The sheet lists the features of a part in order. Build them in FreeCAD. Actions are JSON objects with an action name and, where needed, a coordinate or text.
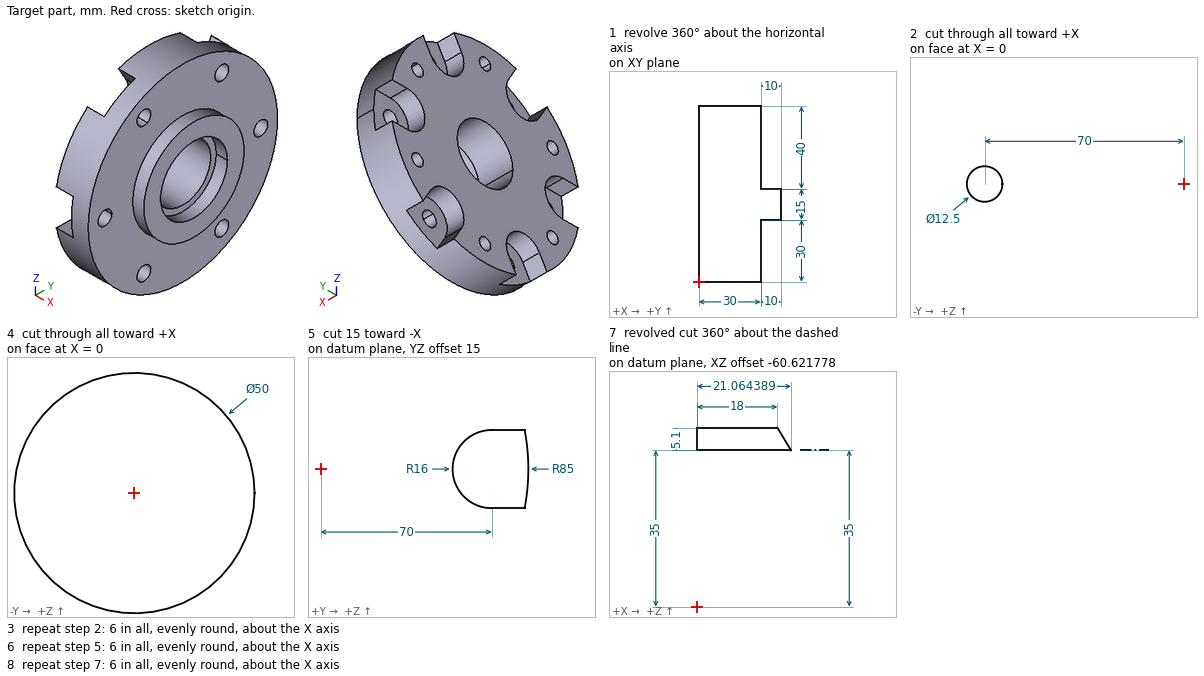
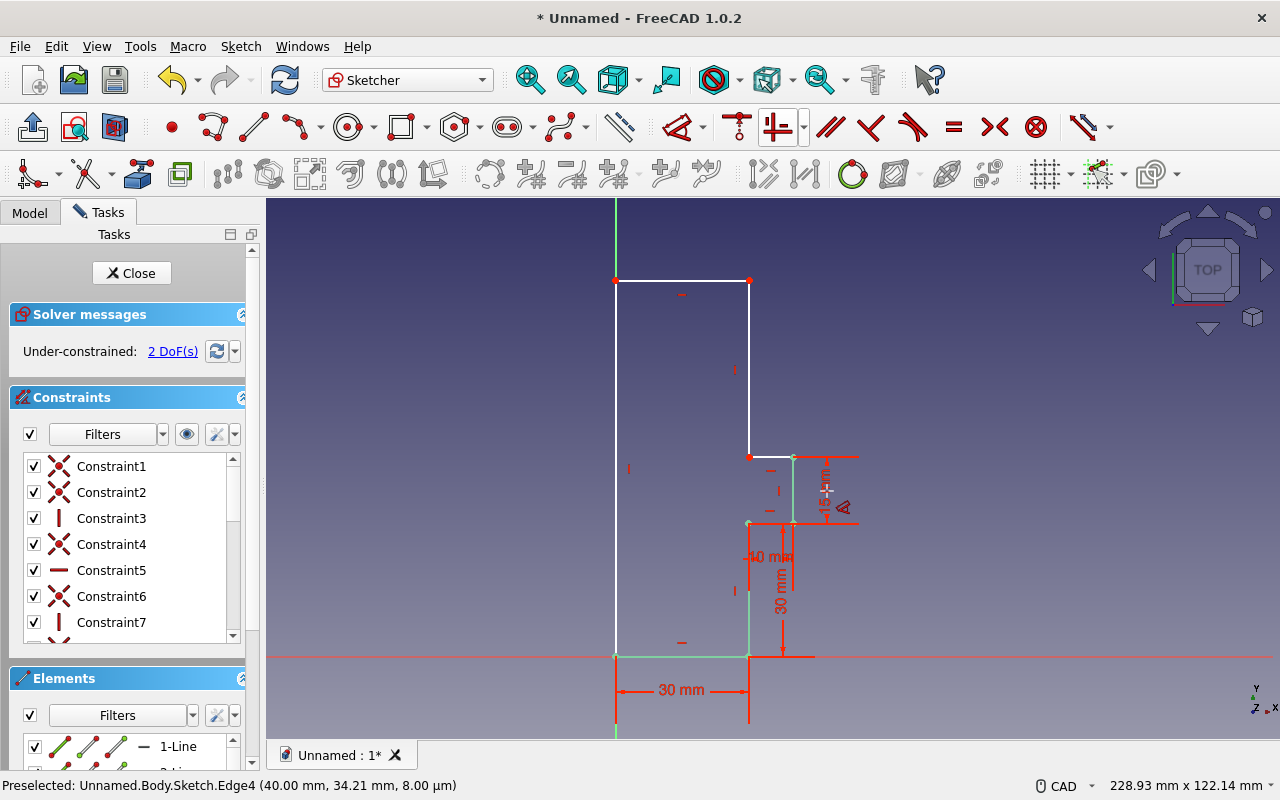
{"action": "left_click", "coordinate": [780, 457]}
{"action": "left_click", "coordinate": [771, 423]}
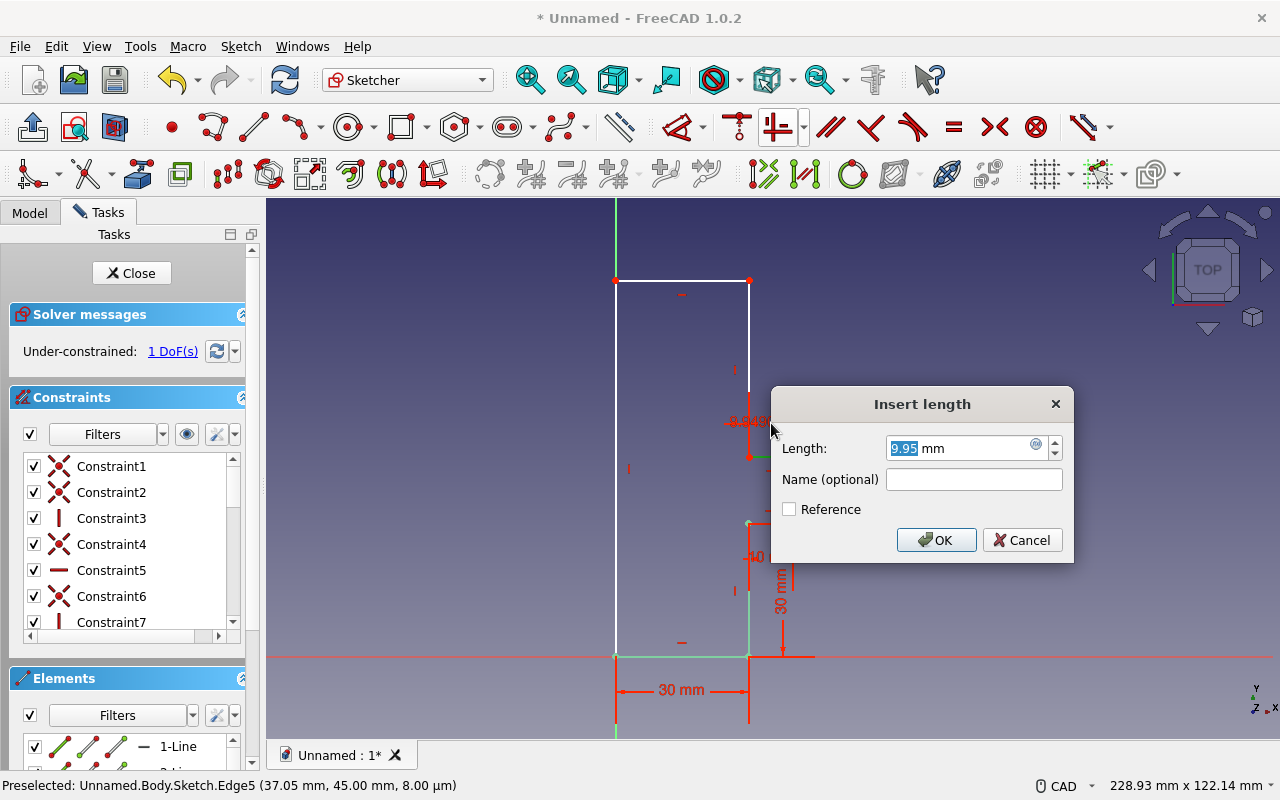
{"action": "type", "text": "10"}
{"action": "key", "text": "Return"}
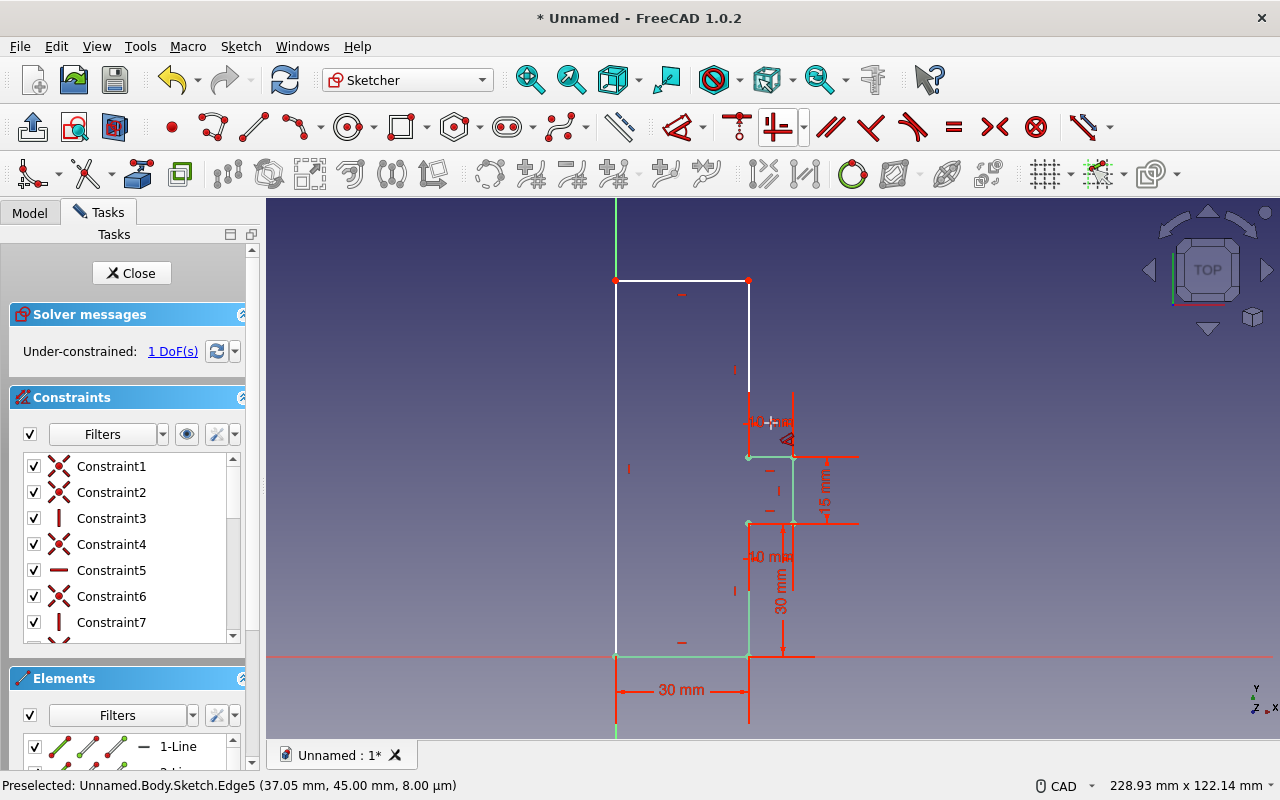
{"action": "left_click", "coordinate": [749, 404]}
{"action": "left_click", "coordinate": [783, 369]}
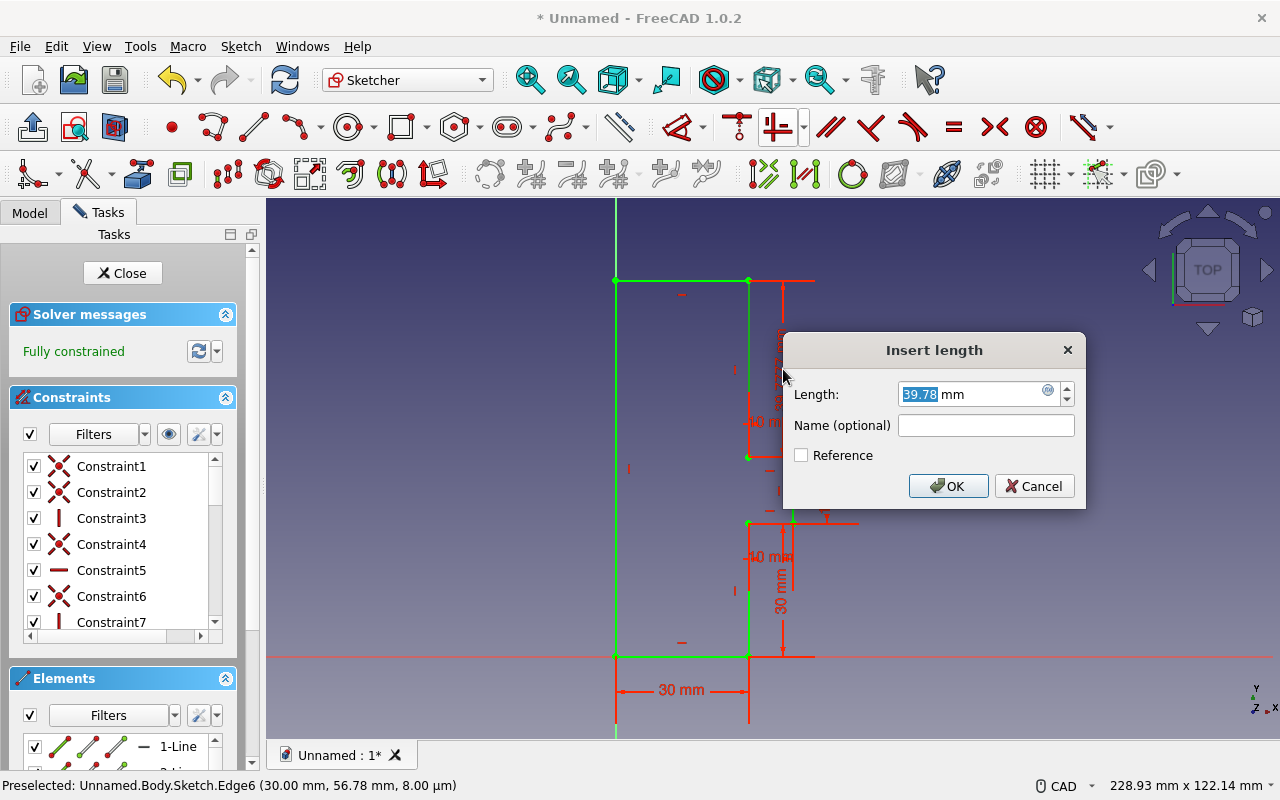
{"action": "type", "text": "40"}
{"action": "key", "text": "Return"}
{"action": "key", "text": "Escape"}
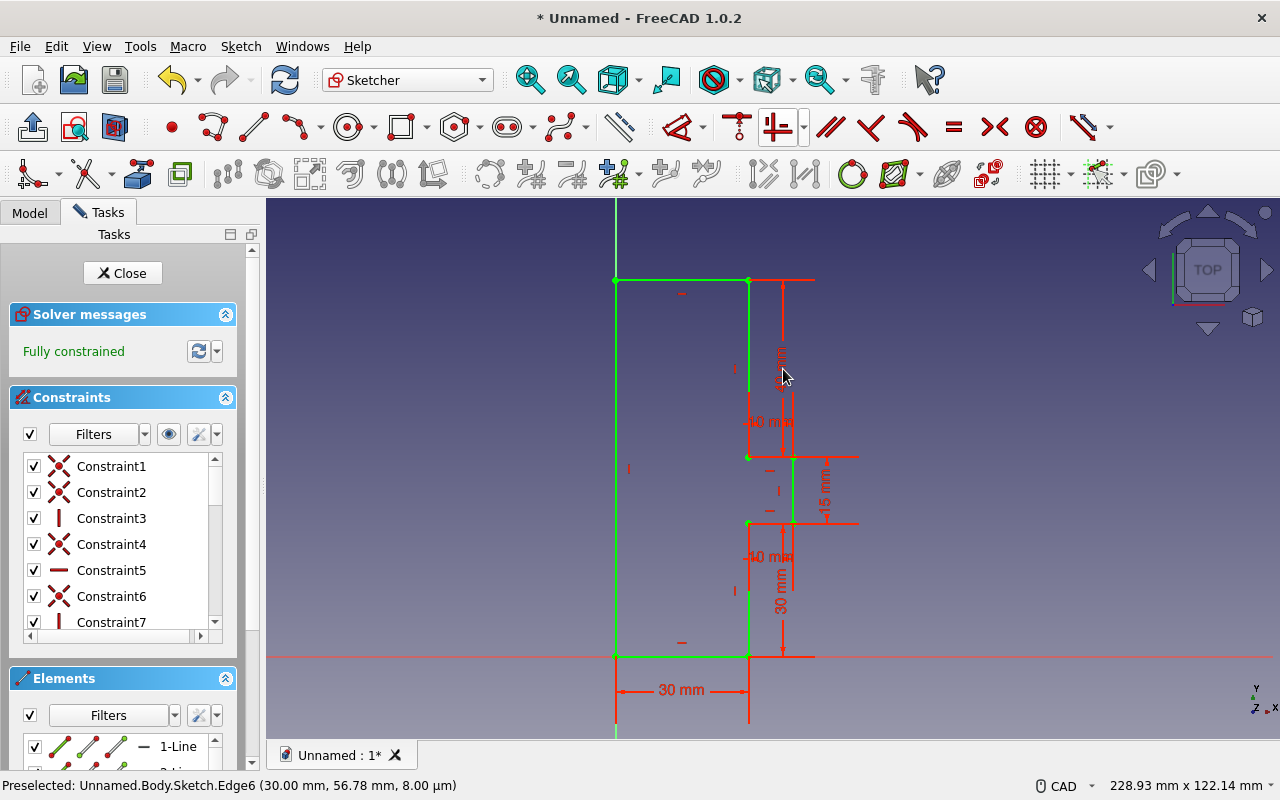
{"action": "left_click", "coordinate": [123, 273]}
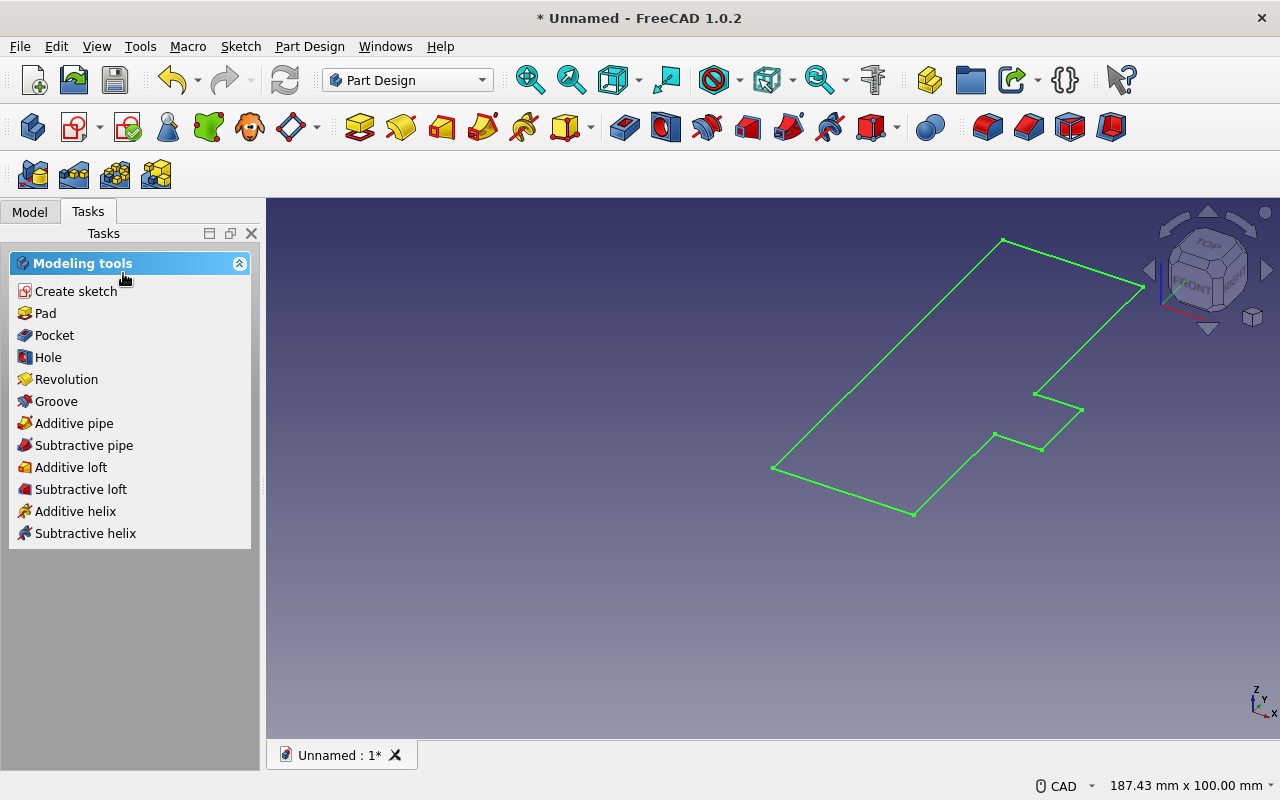
{"action": "left_click", "coordinate": [401, 128]}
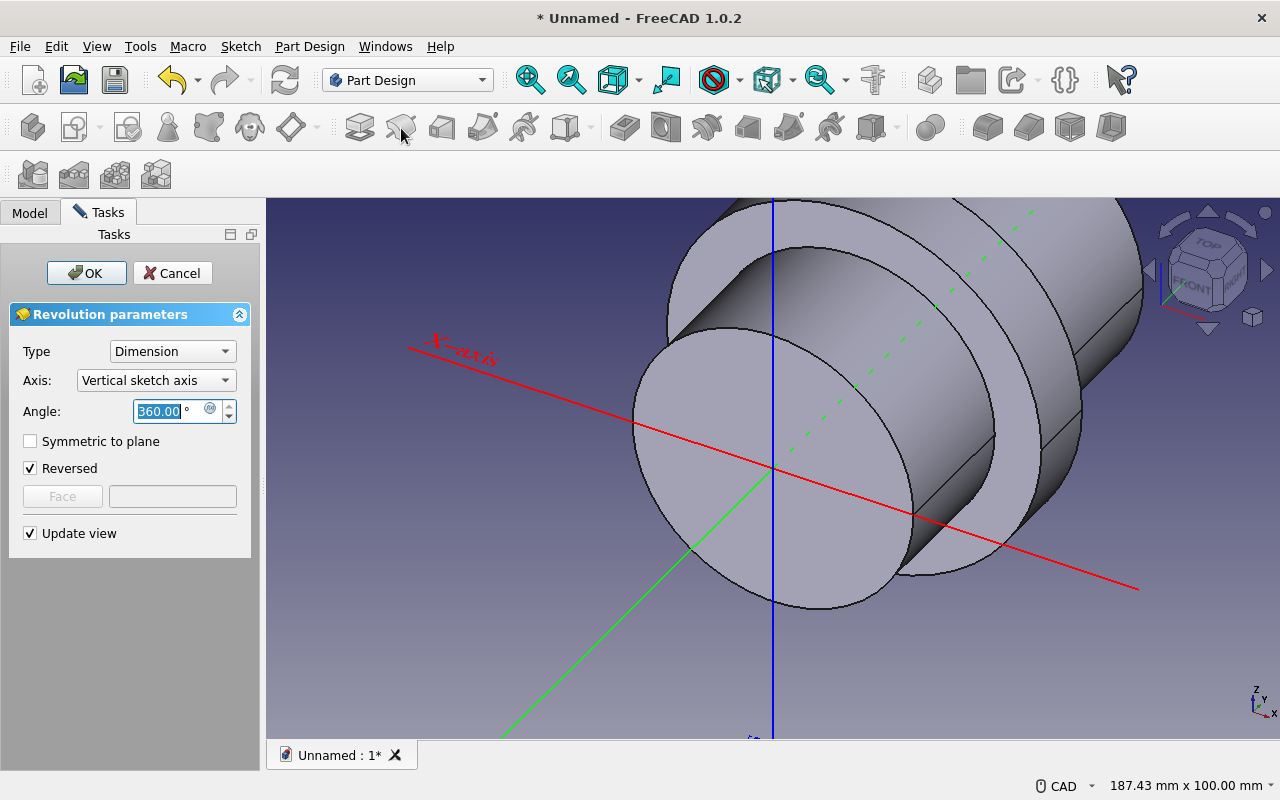
{"action": "left_click", "coordinate": [157, 380]}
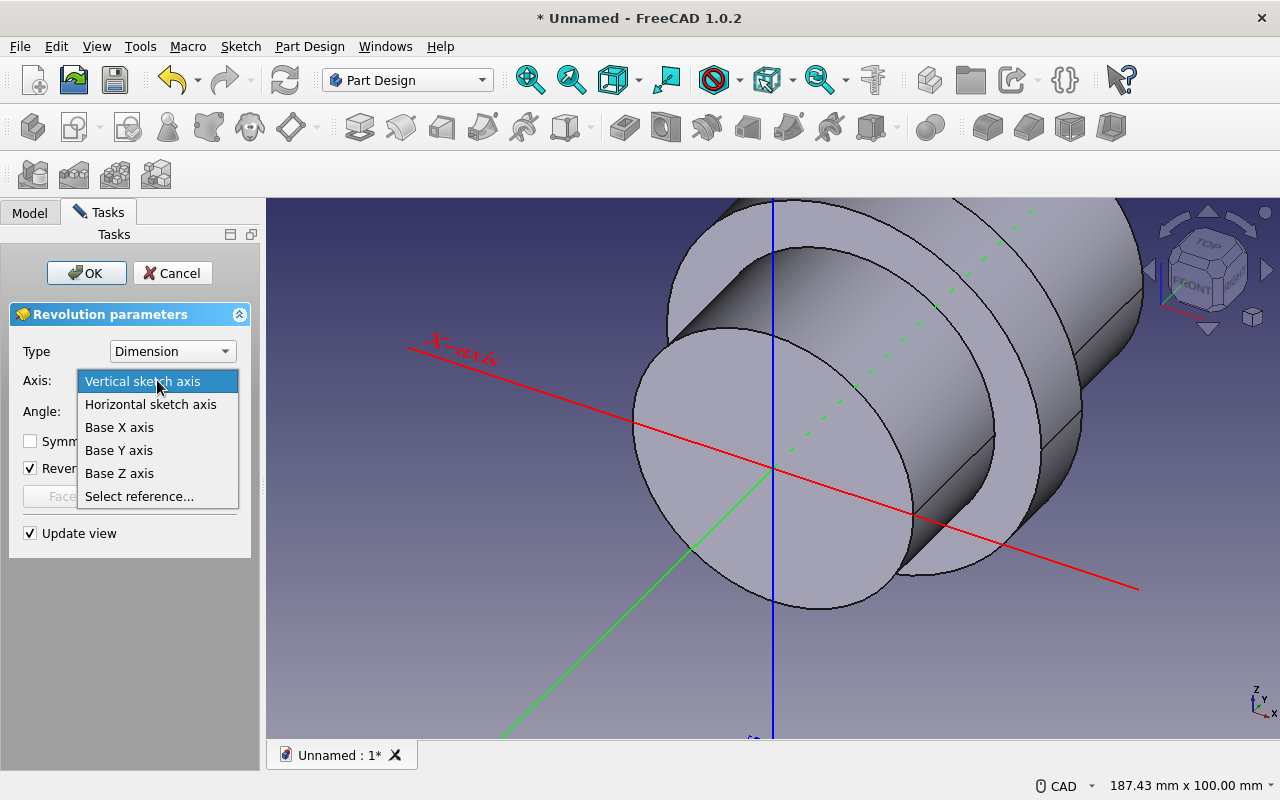
{"action": "left_click", "coordinate": [156, 404]}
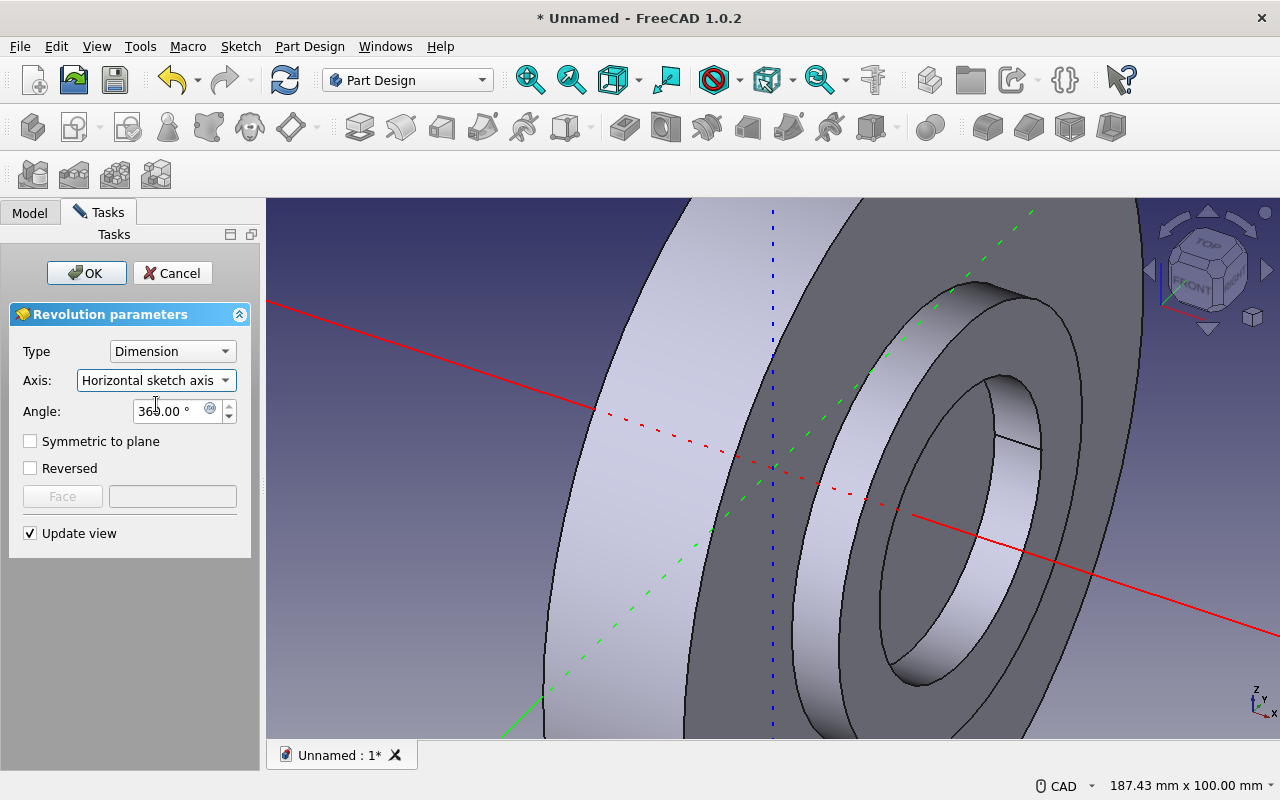
{"action": "left_click", "coordinate": [87, 273]}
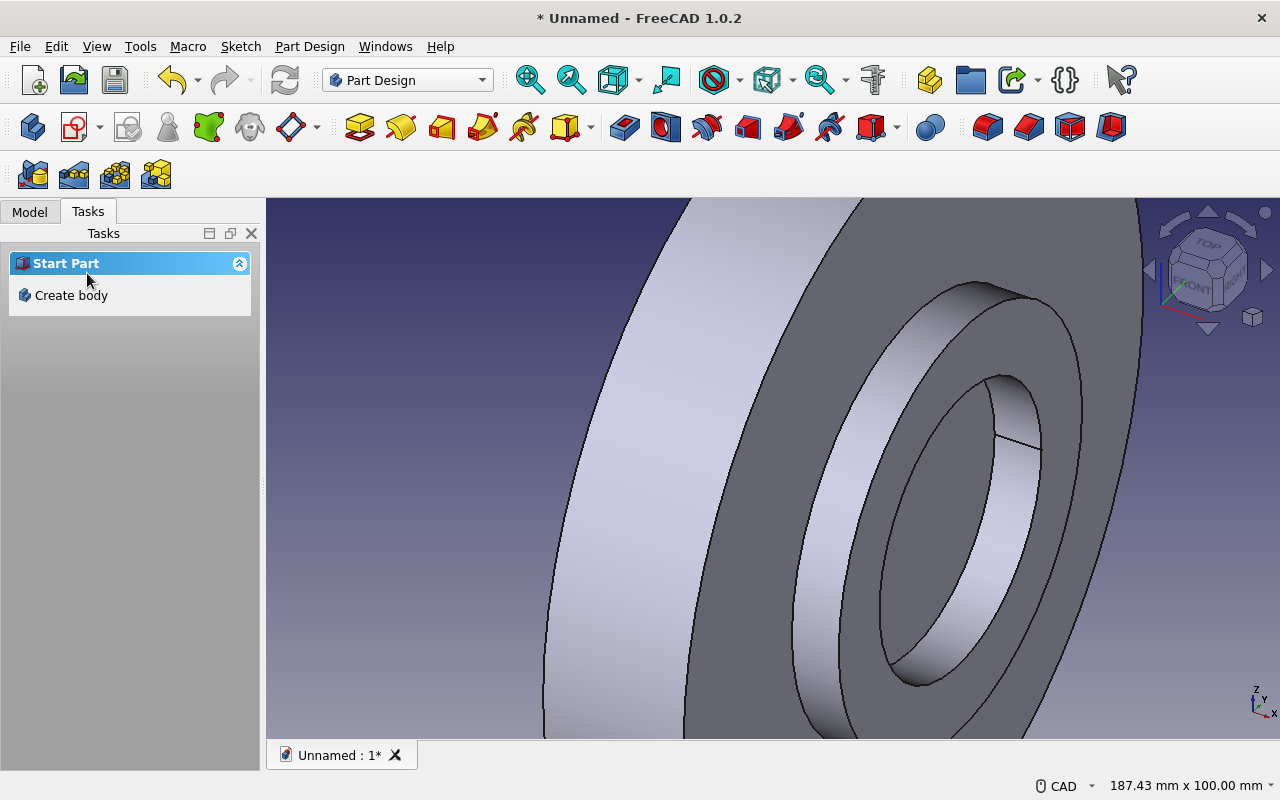
{"action": "left_click", "coordinate": [531, 80]}